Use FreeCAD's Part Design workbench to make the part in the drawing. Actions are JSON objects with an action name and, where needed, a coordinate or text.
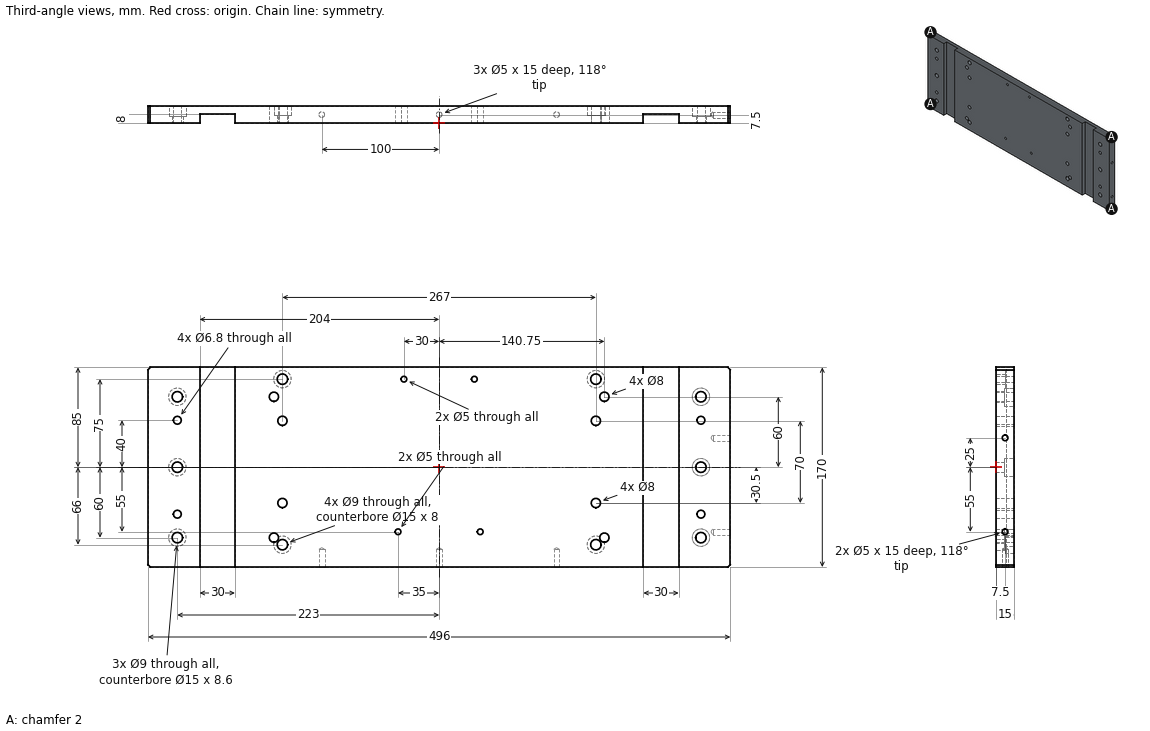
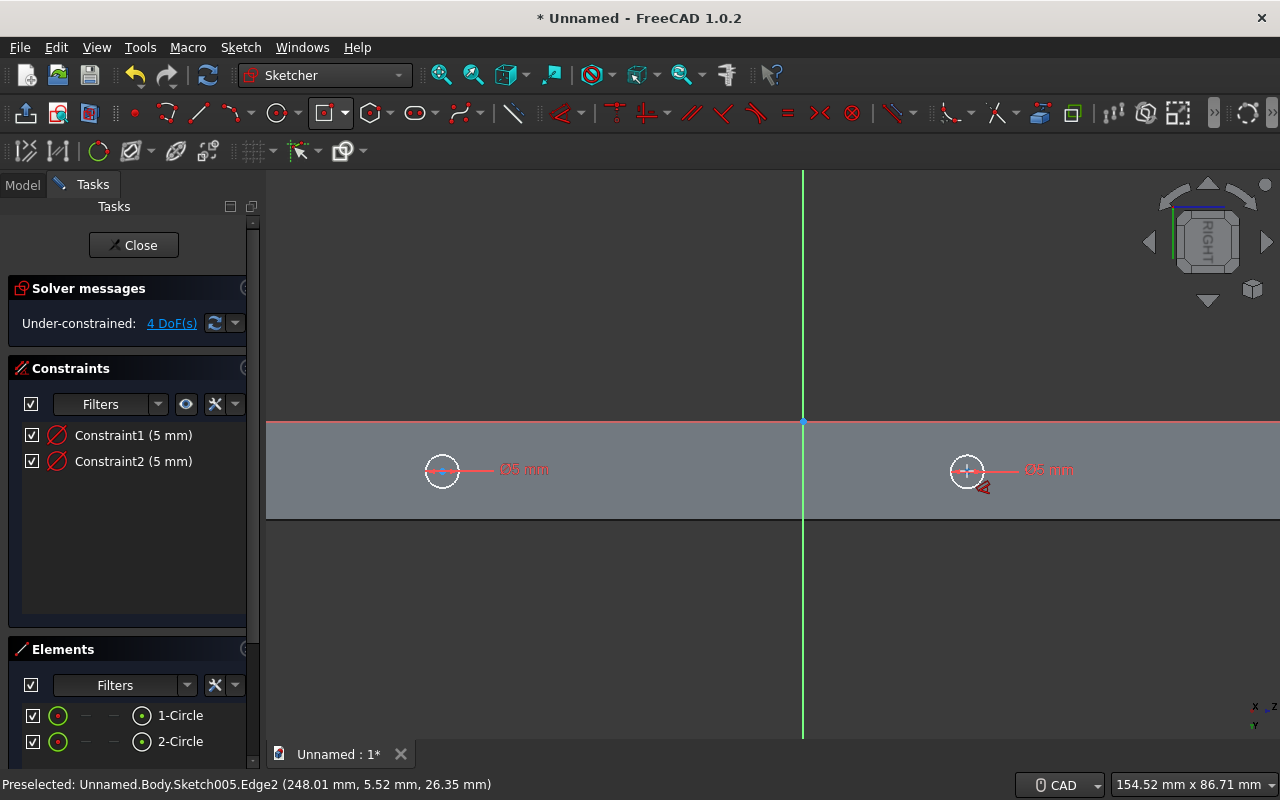
{"action": "left_click", "coordinate": [442, 471]}
{"action": "left_click", "coordinate": [623, 388]}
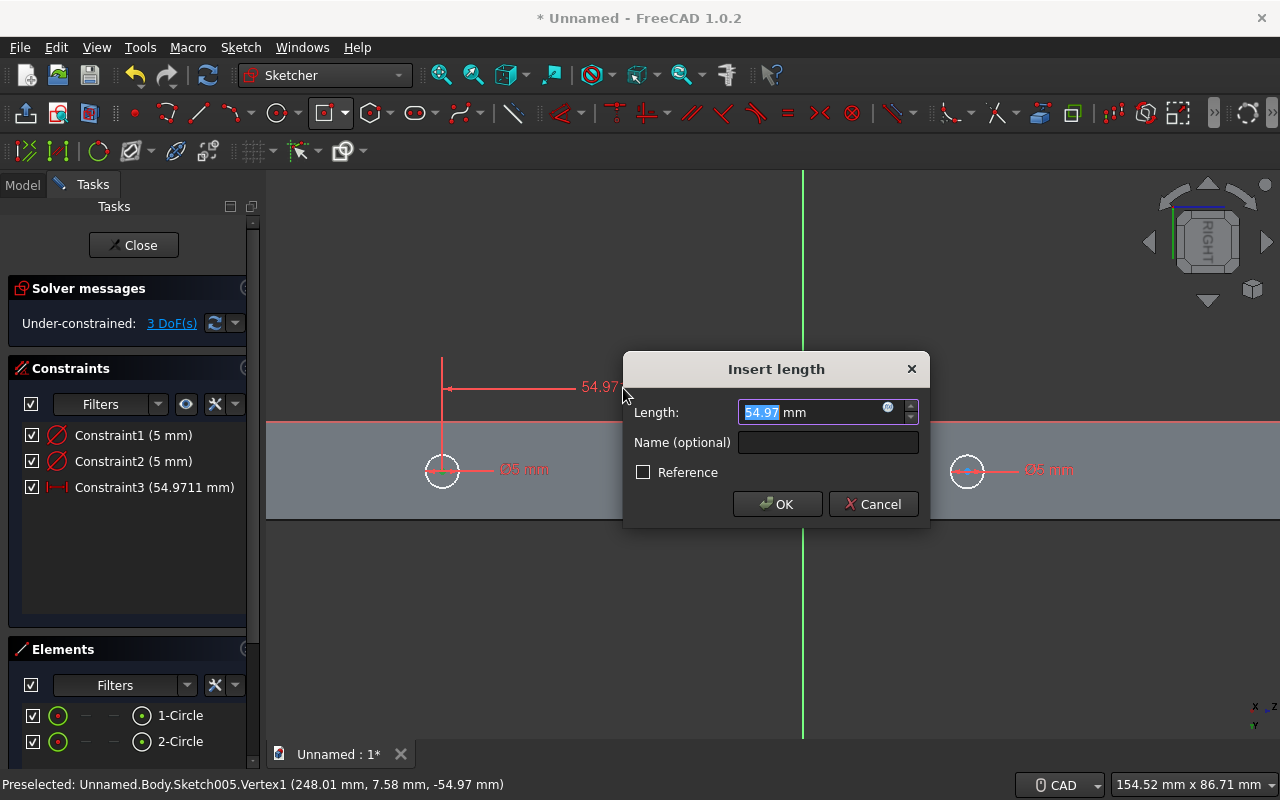
{"action": "type", "text": "55"}
{"action": "key", "text": "Return"}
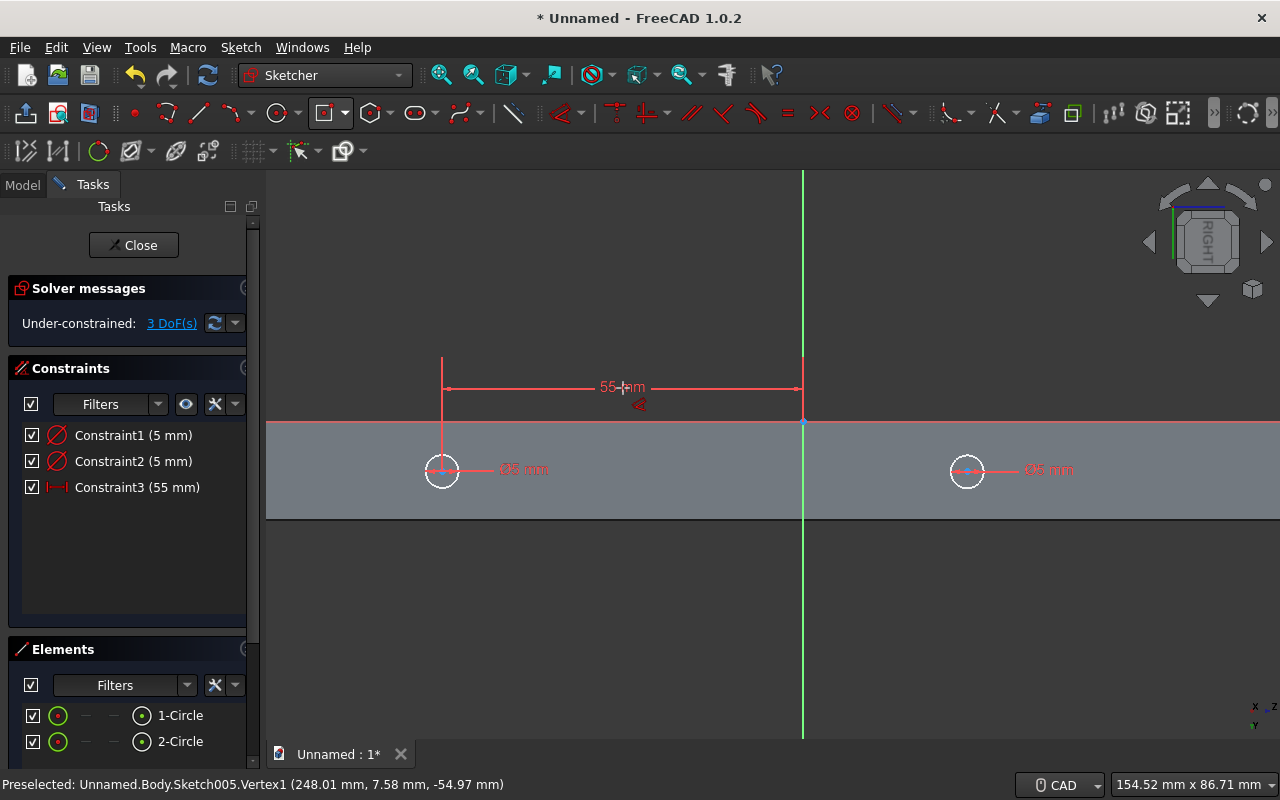
{"action": "left_click", "coordinate": [967, 472]}
{"action": "left_click", "coordinate": [885, 388]}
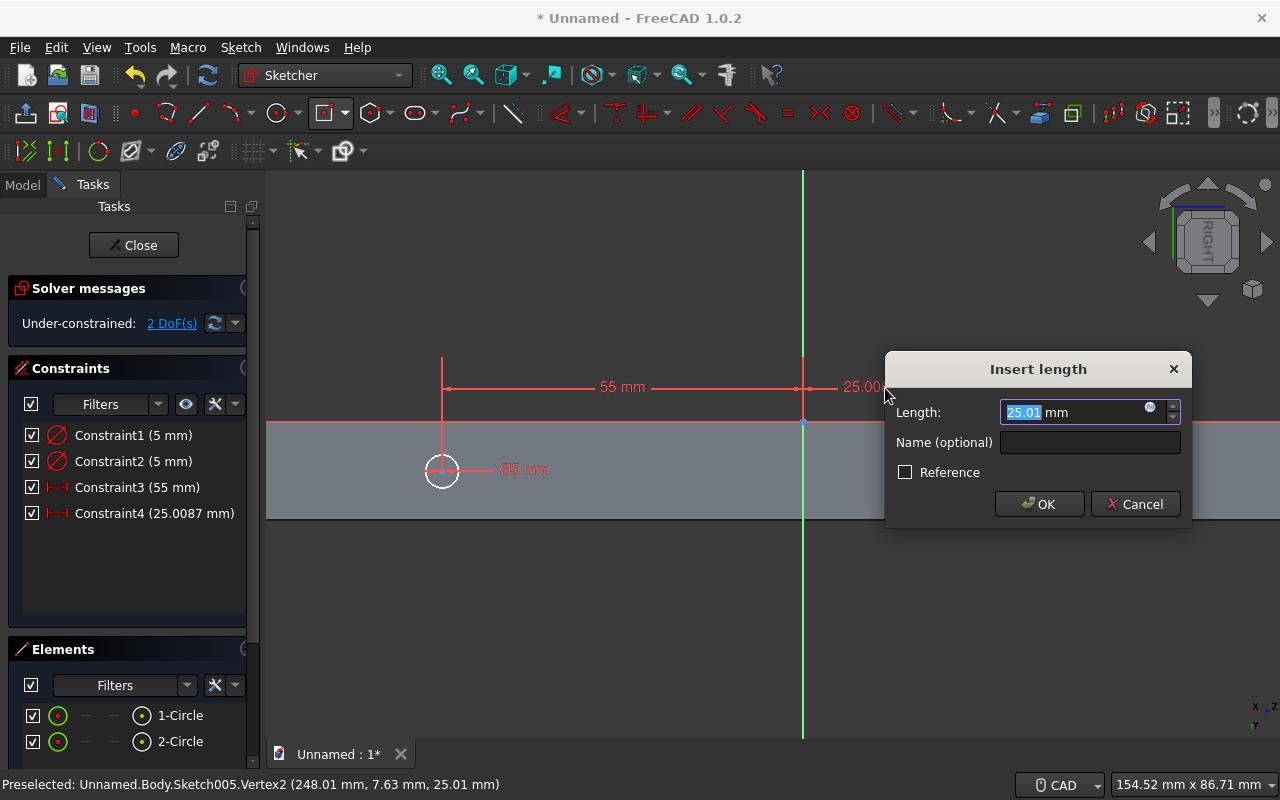
{"action": "type", "text": "25"}
{"action": "key", "text": "Return"}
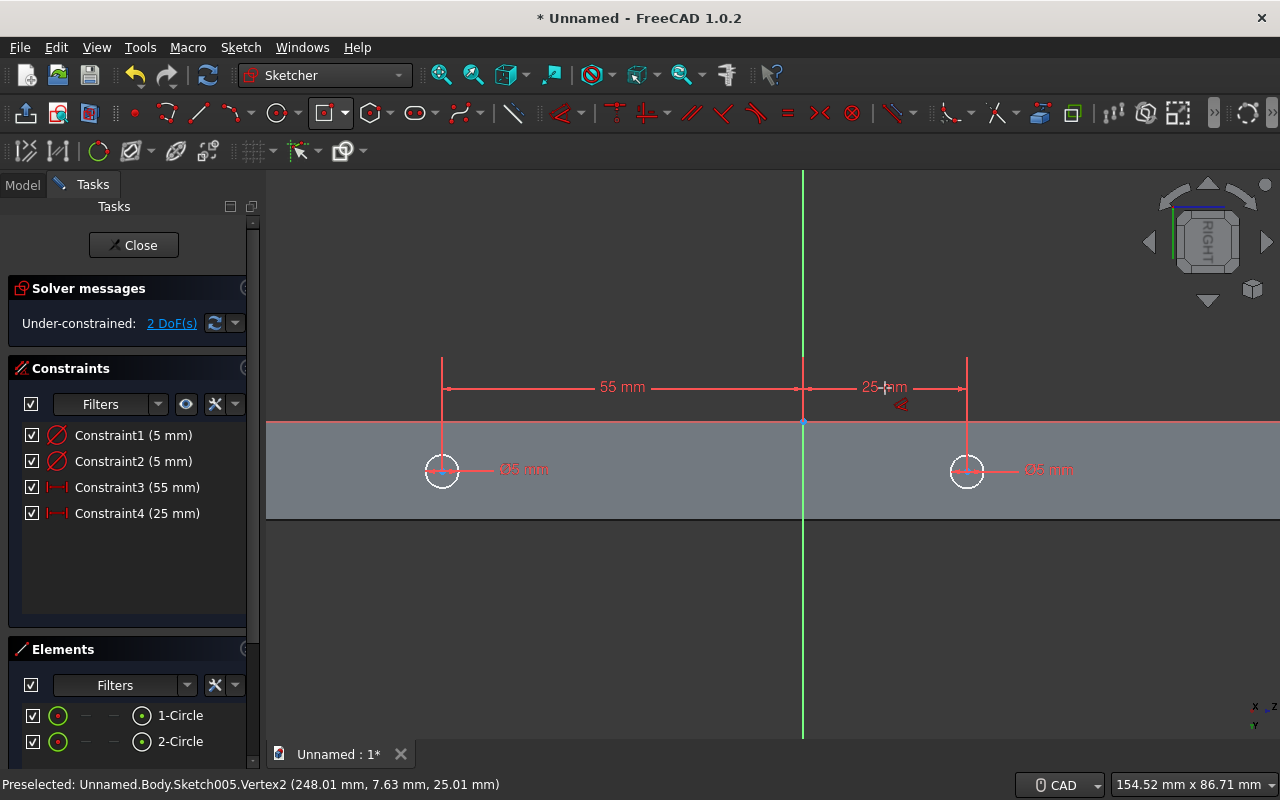
{"action": "left_click", "coordinate": [442, 471]}
{"action": "left_click", "coordinate": [408, 447]}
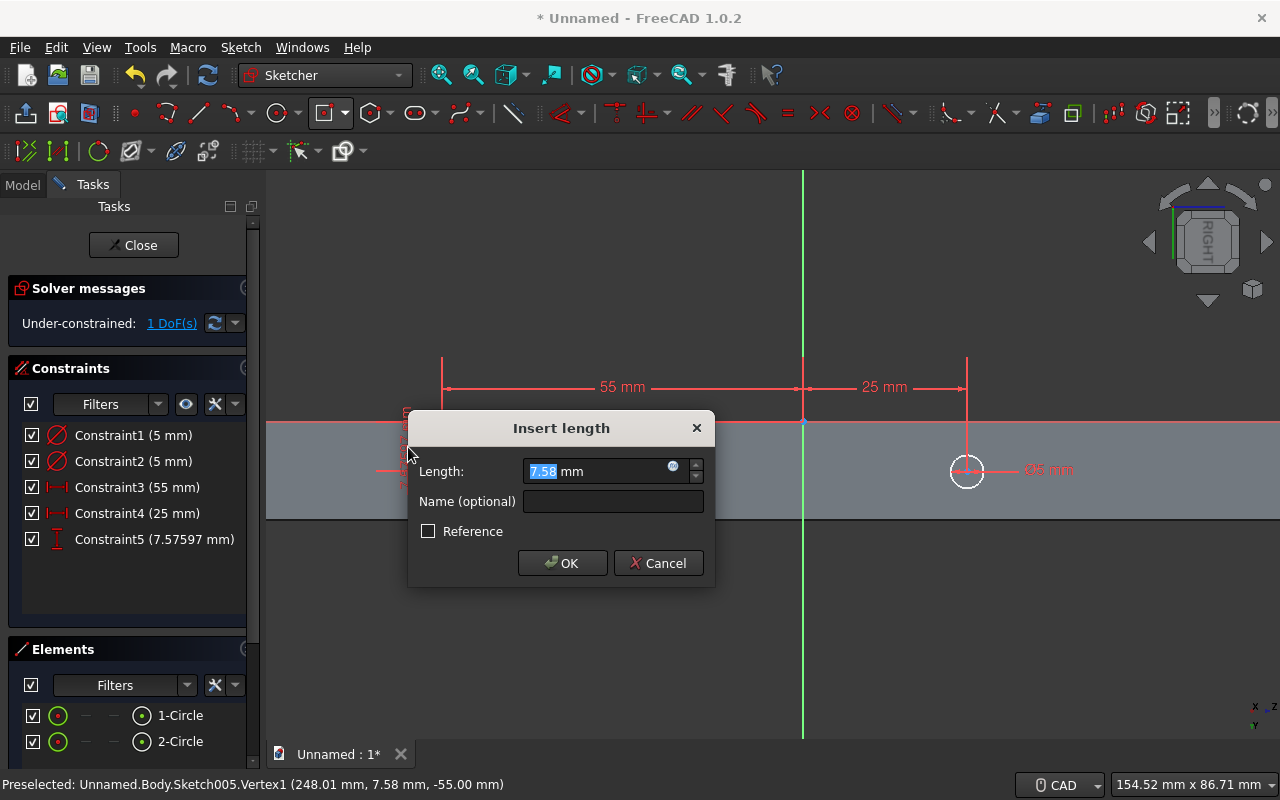
{"action": "type", "text": "7.5"}
{"action": "key", "text": "Return"}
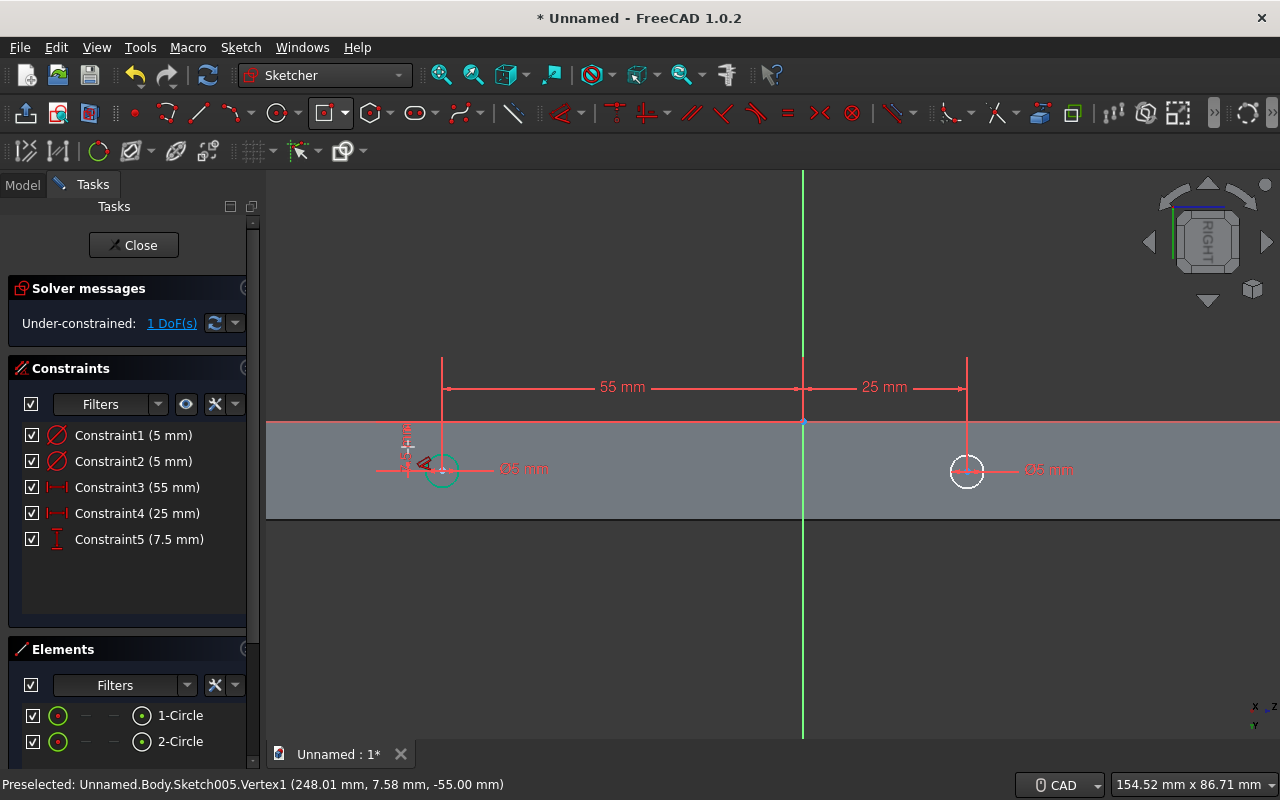
{"action": "left_click", "coordinate": [967, 472]}
{"action": "left_click", "coordinate": [1001, 447]}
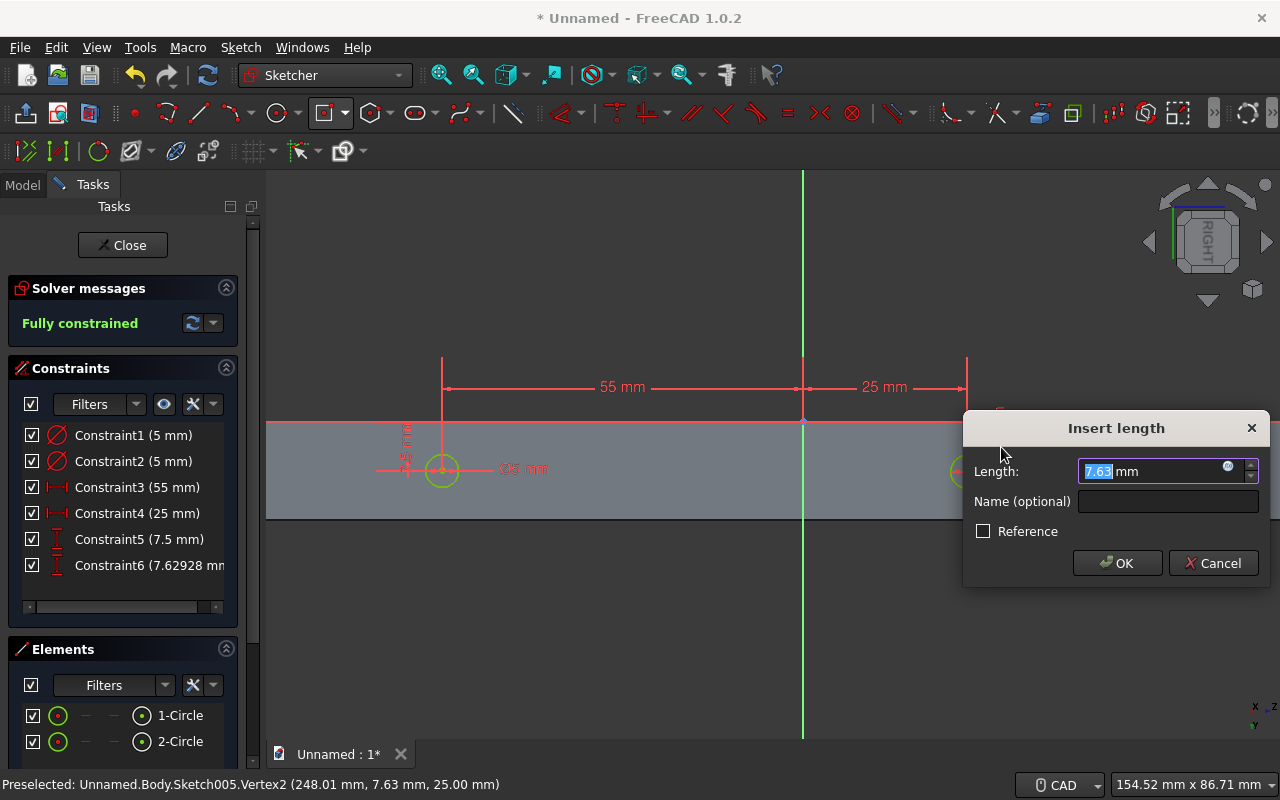
{"action": "type", "text": "7.5"}
{"action": "key", "text": "Return"}
{"action": "key", "text": "Escape"}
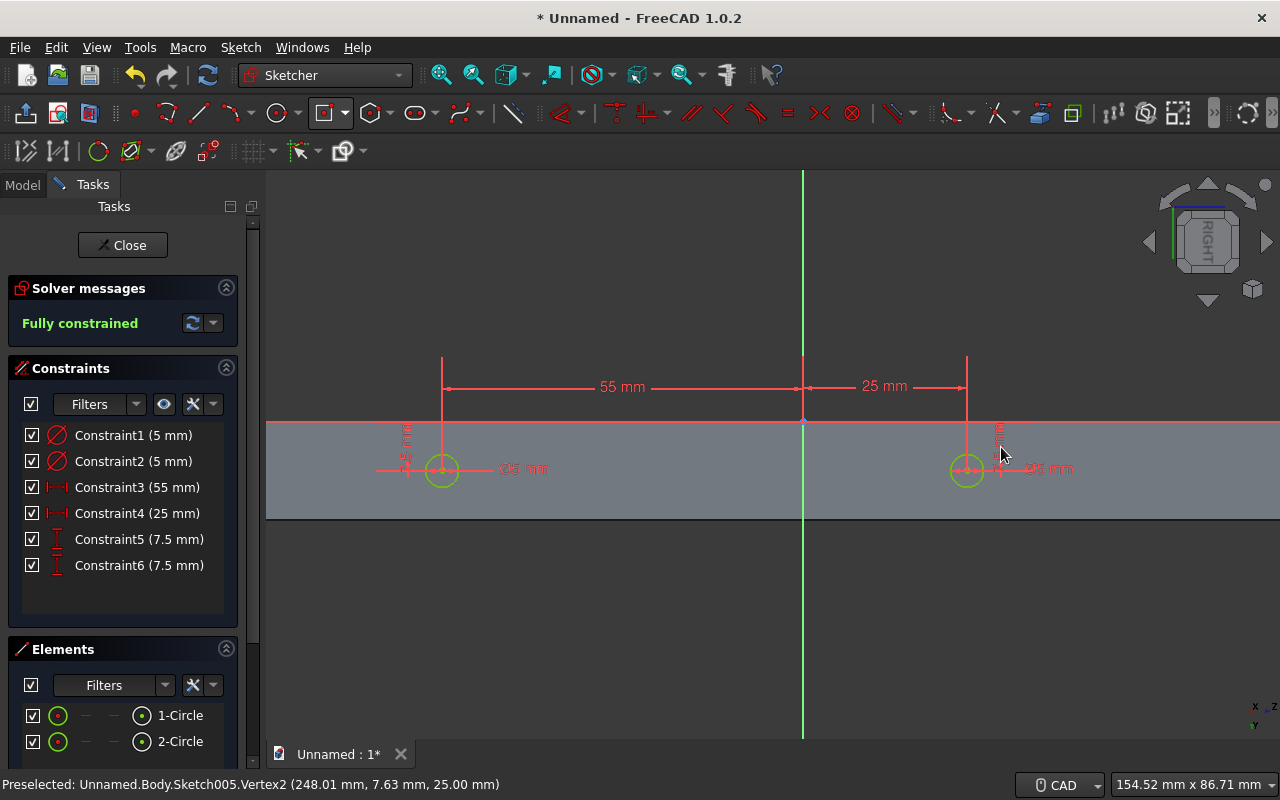
{"action": "left_click", "coordinate": [123, 245]}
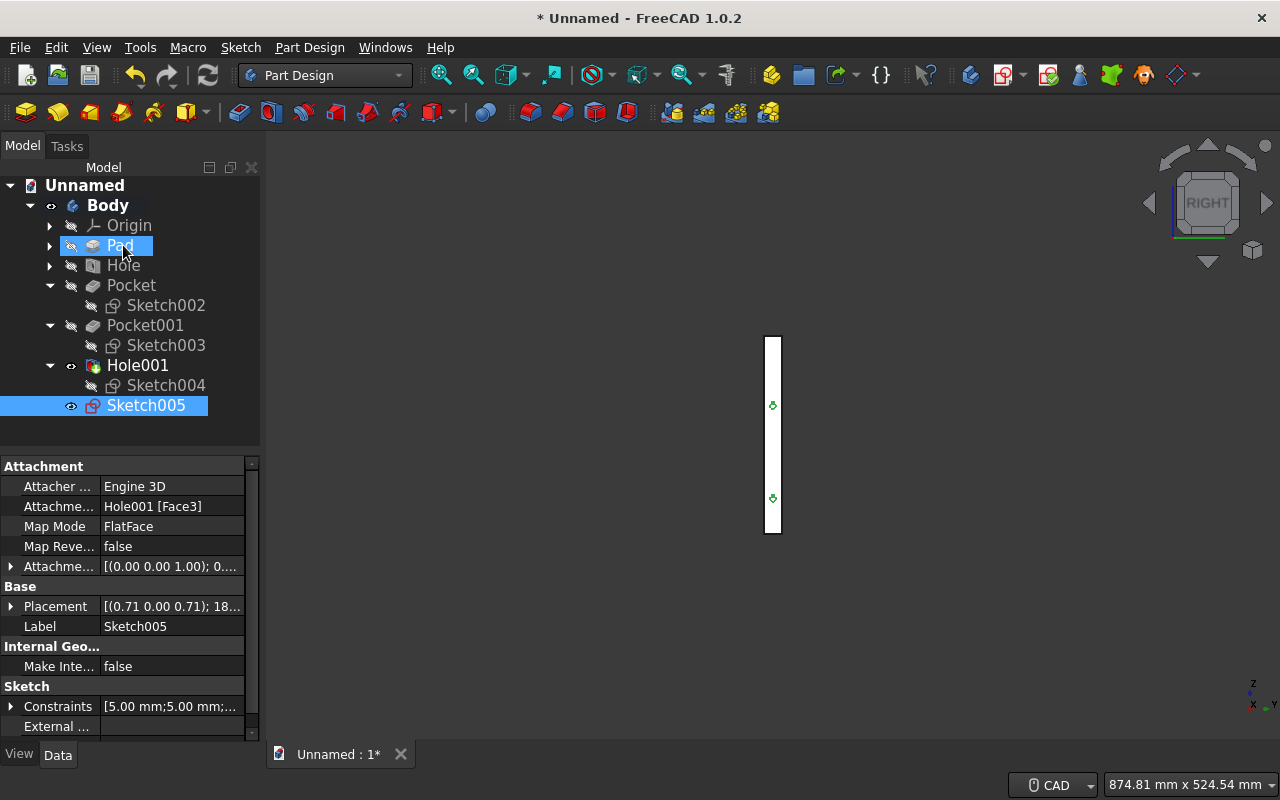
{"action": "left_click", "coordinate": [272, 112]}